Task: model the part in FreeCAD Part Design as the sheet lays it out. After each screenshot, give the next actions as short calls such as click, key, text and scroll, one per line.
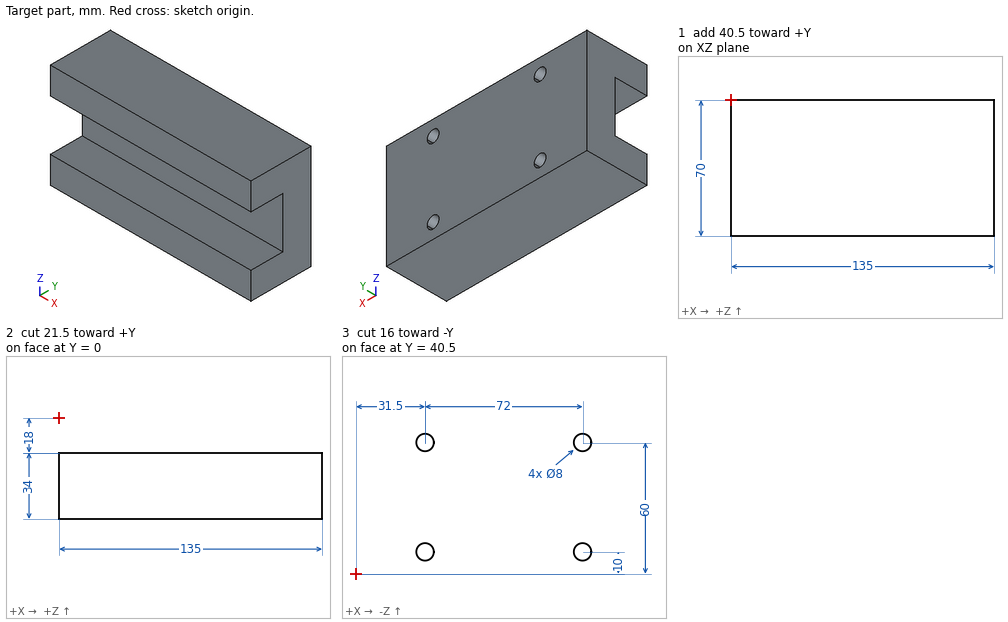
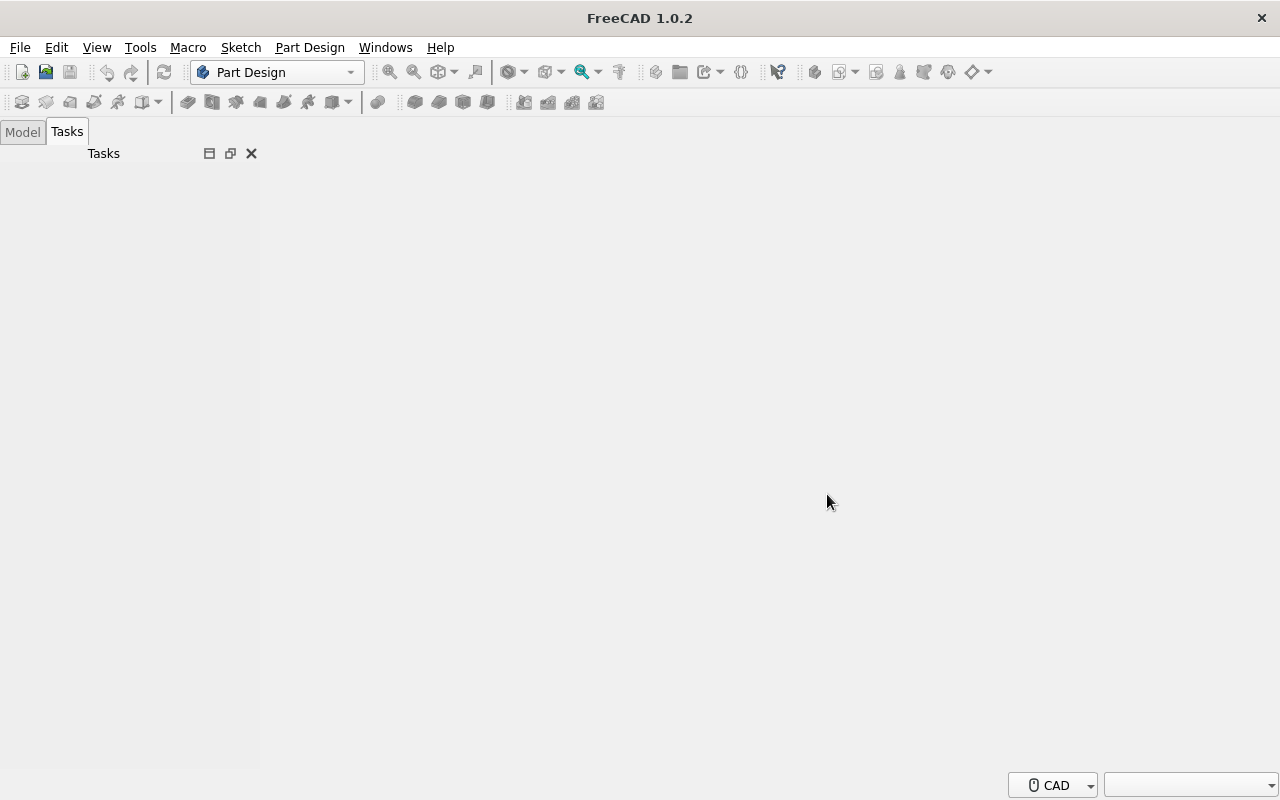
click(22, 72)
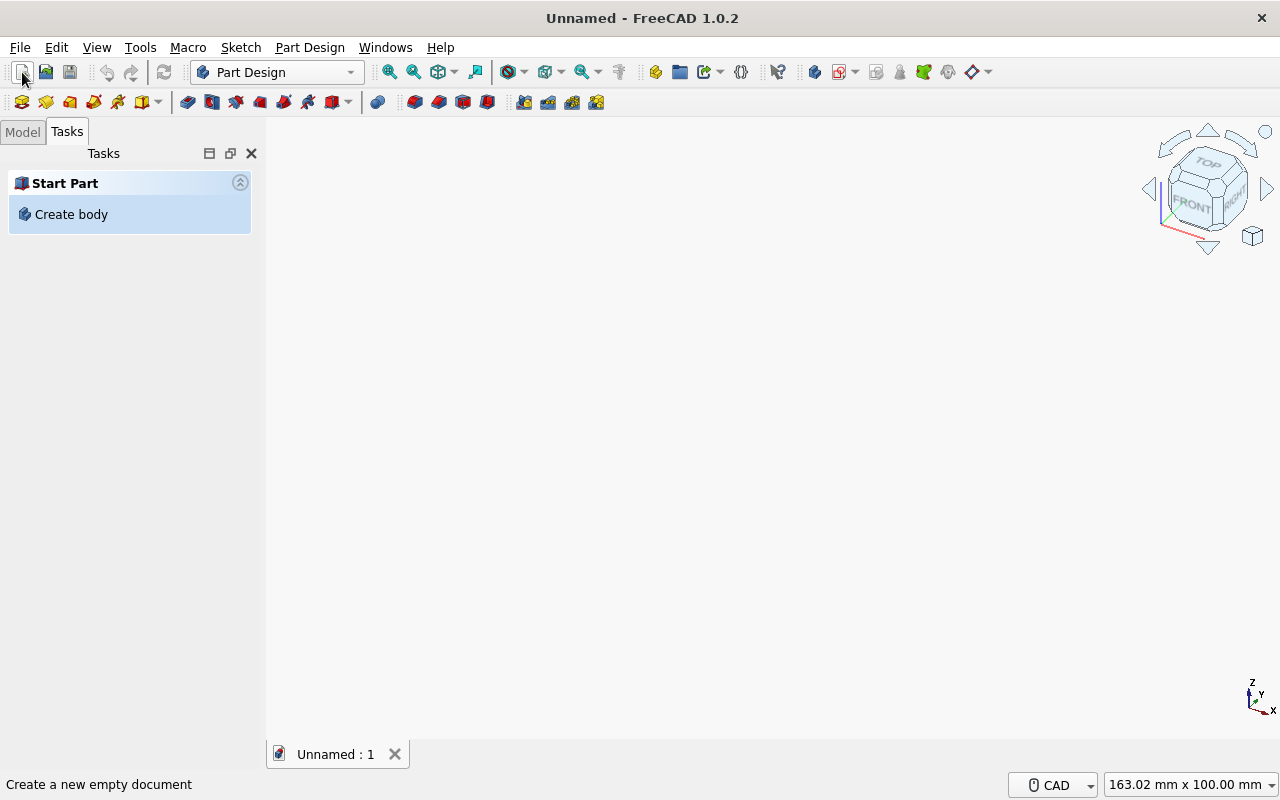
click(840, 72)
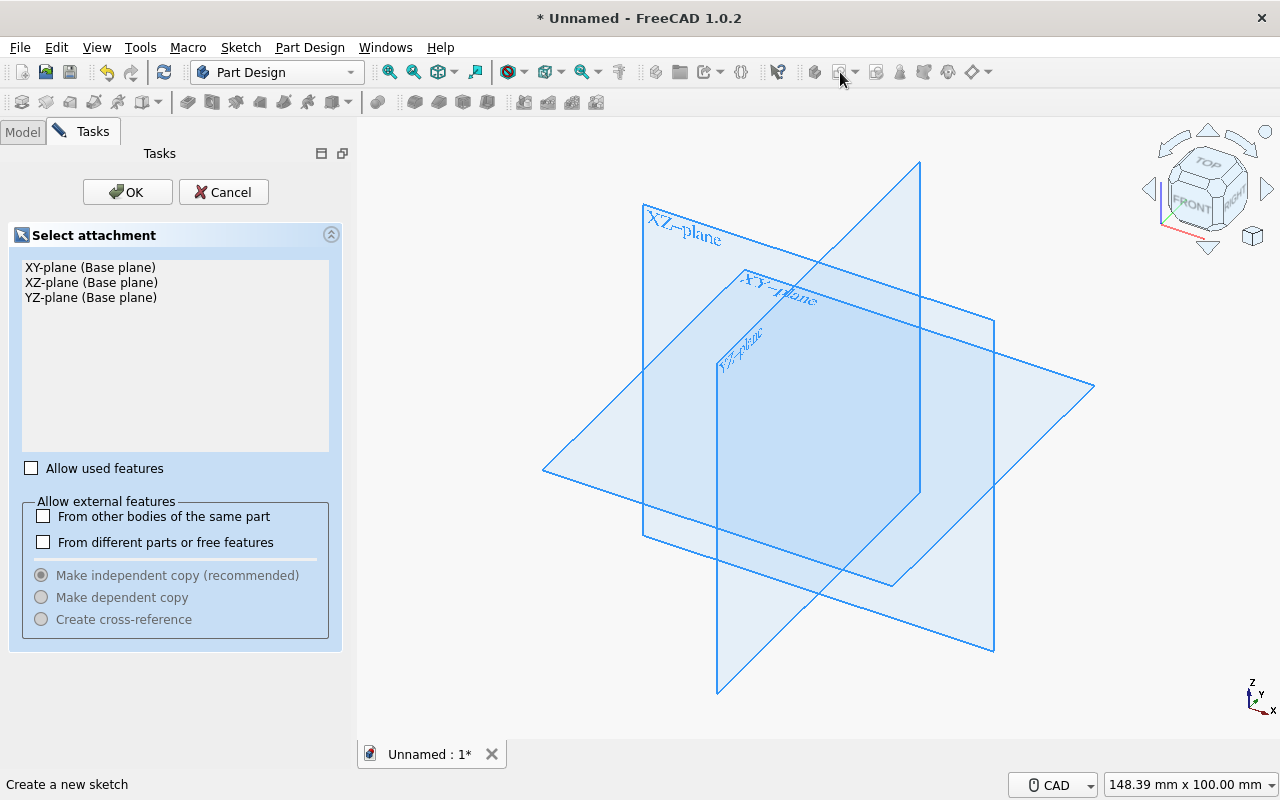
click(82, 282)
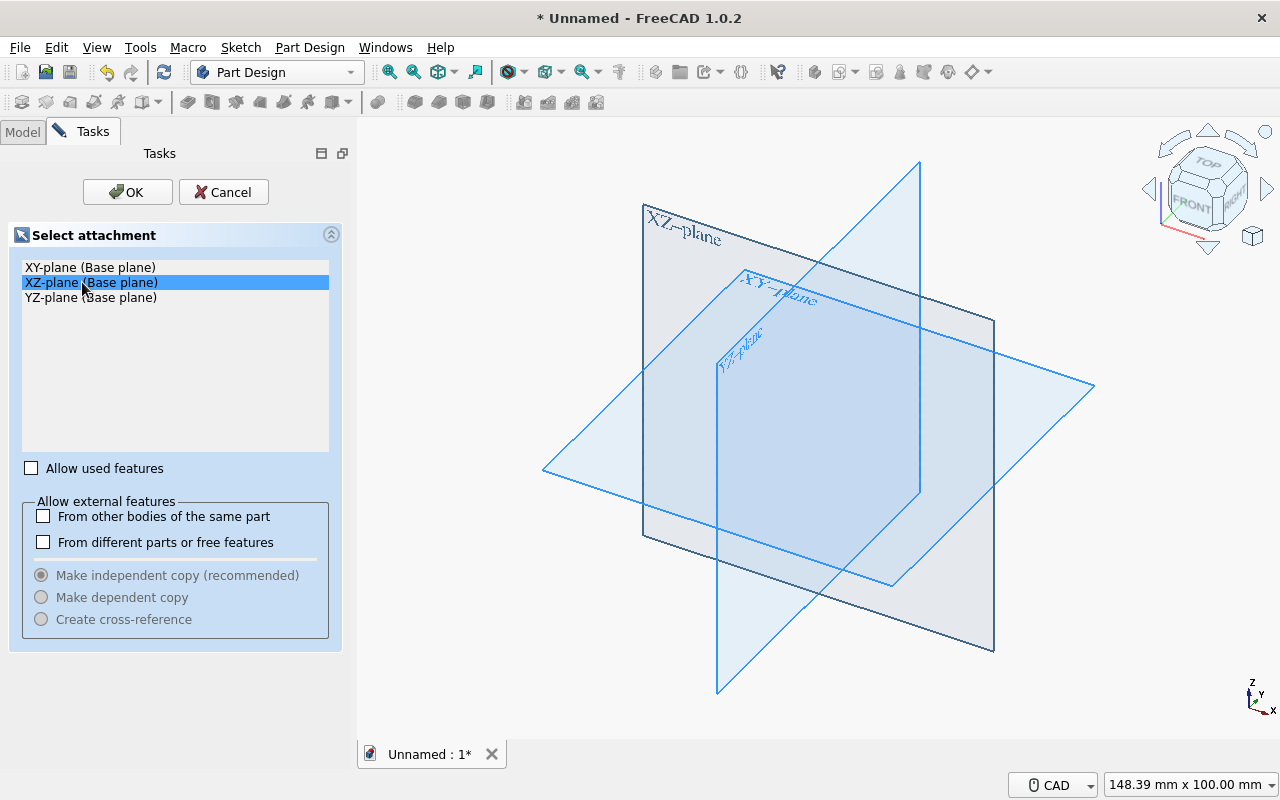
click(128, 192)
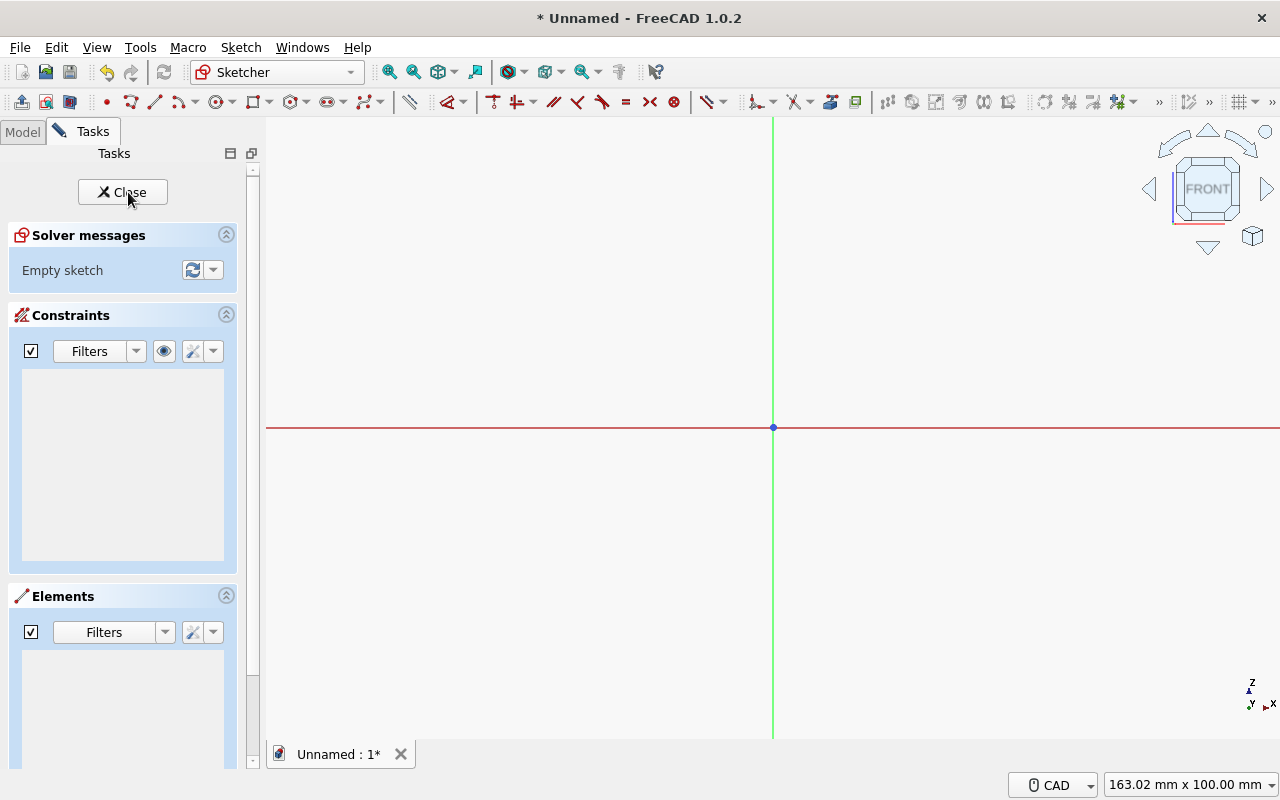
scroll(294, 163, down, 3)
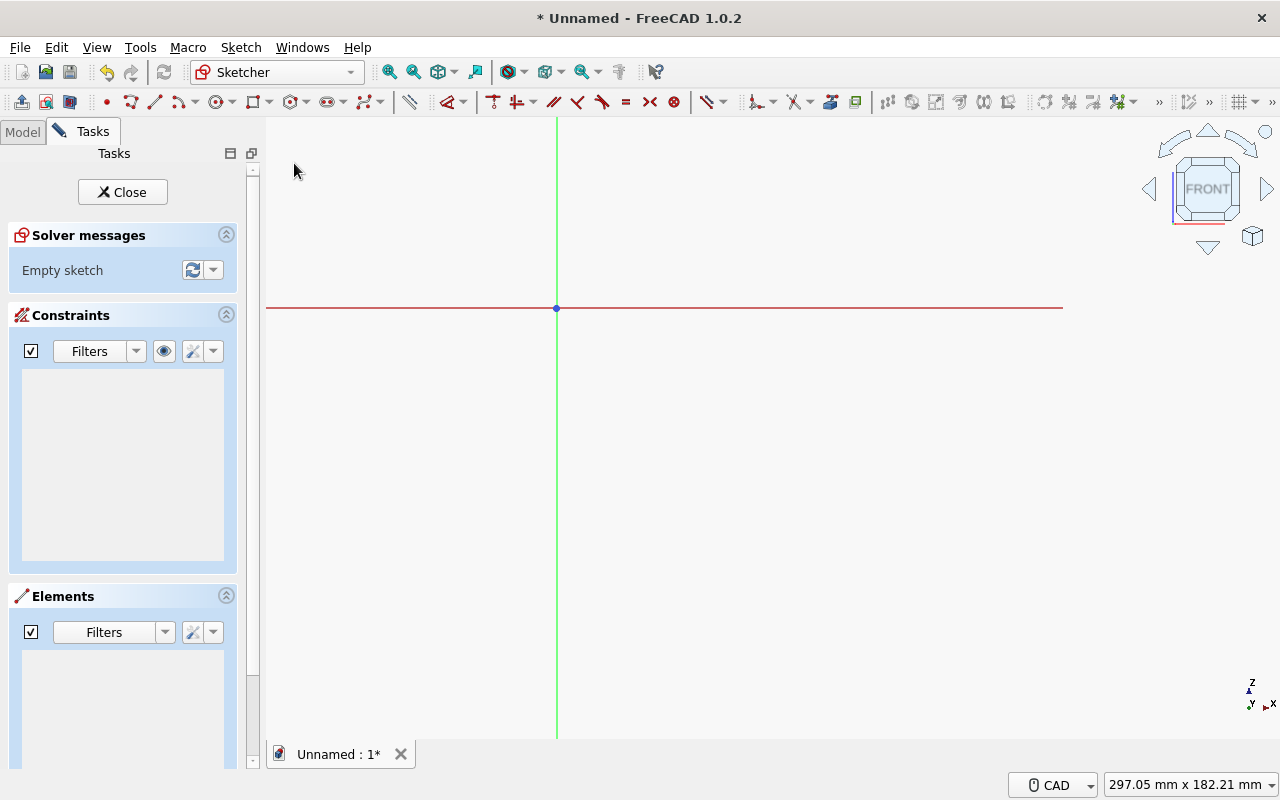
click(254, 102)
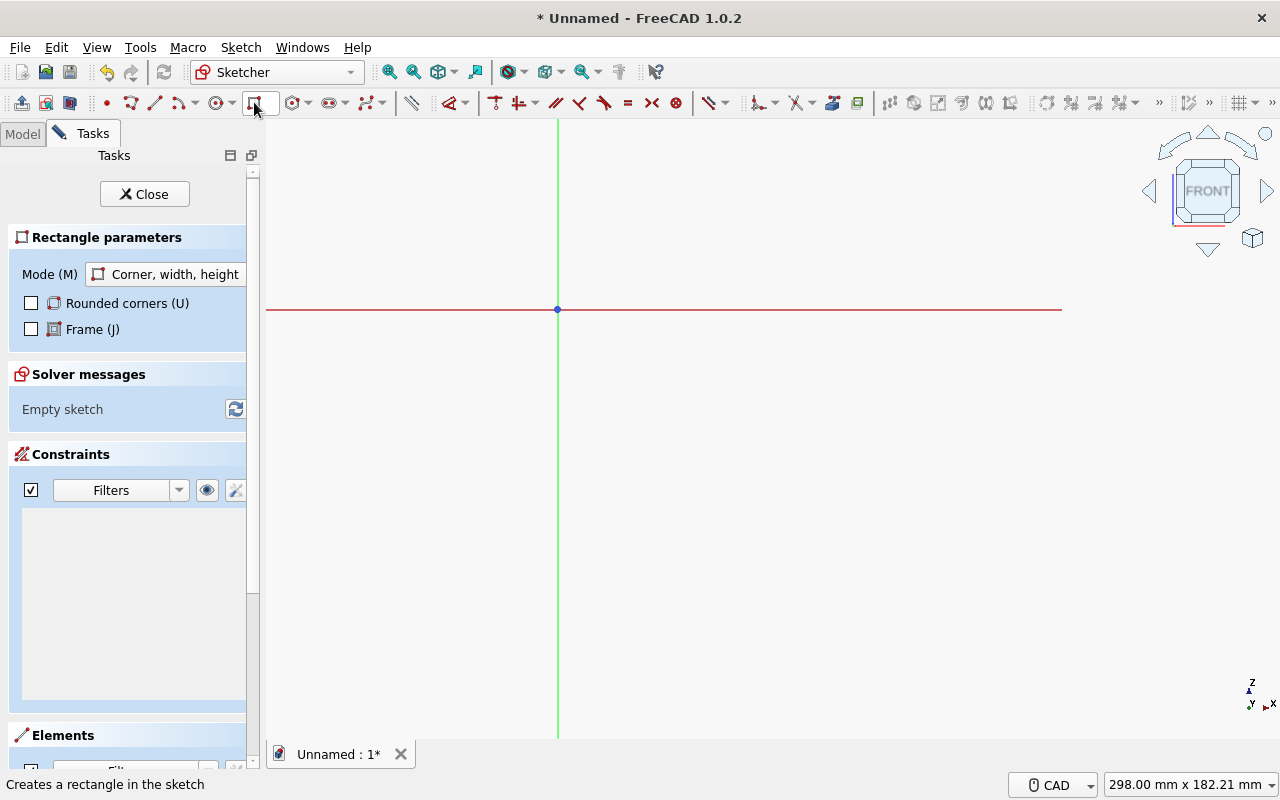
click(558, 310)
click(1017, 548)
key(Escape)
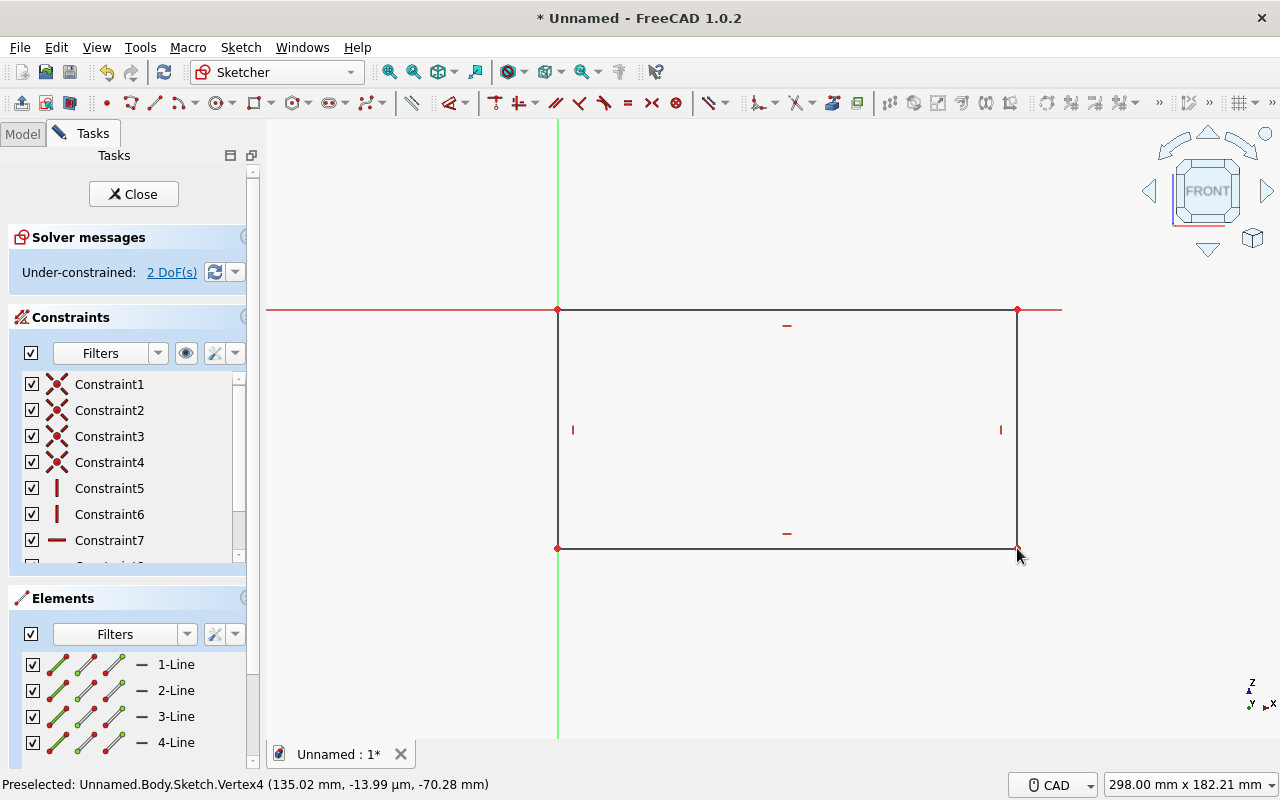
click(558, 382)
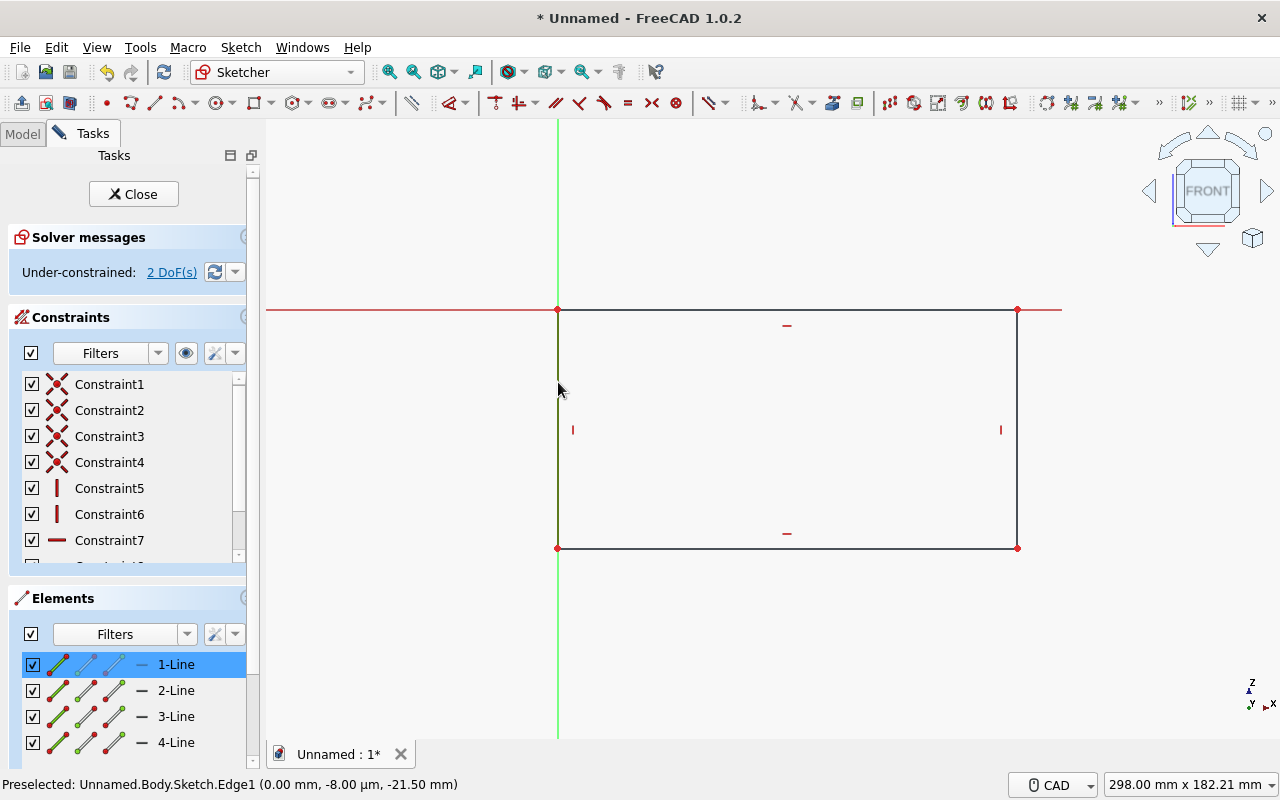
key(i)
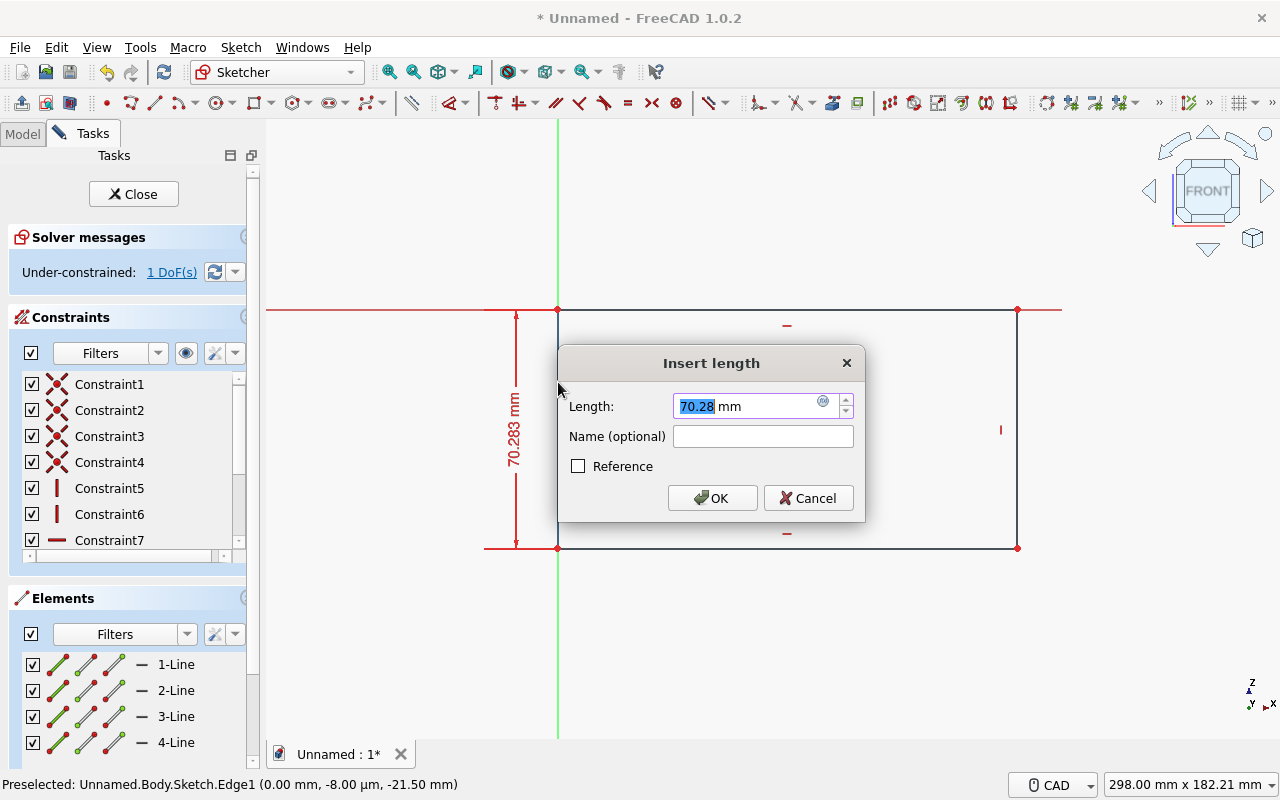
text(70)
key(Return)